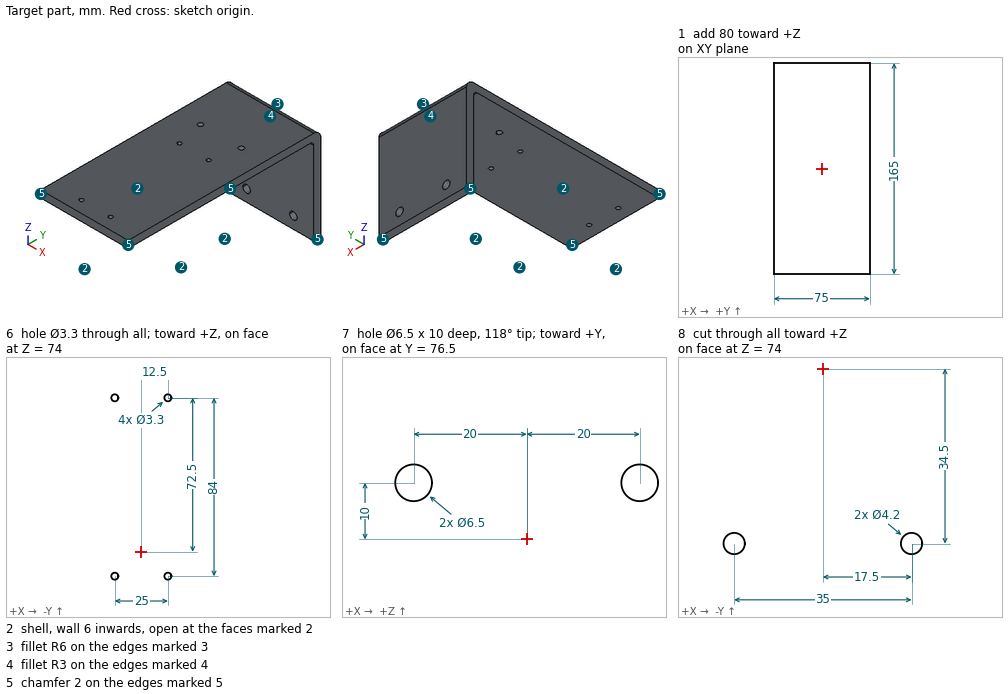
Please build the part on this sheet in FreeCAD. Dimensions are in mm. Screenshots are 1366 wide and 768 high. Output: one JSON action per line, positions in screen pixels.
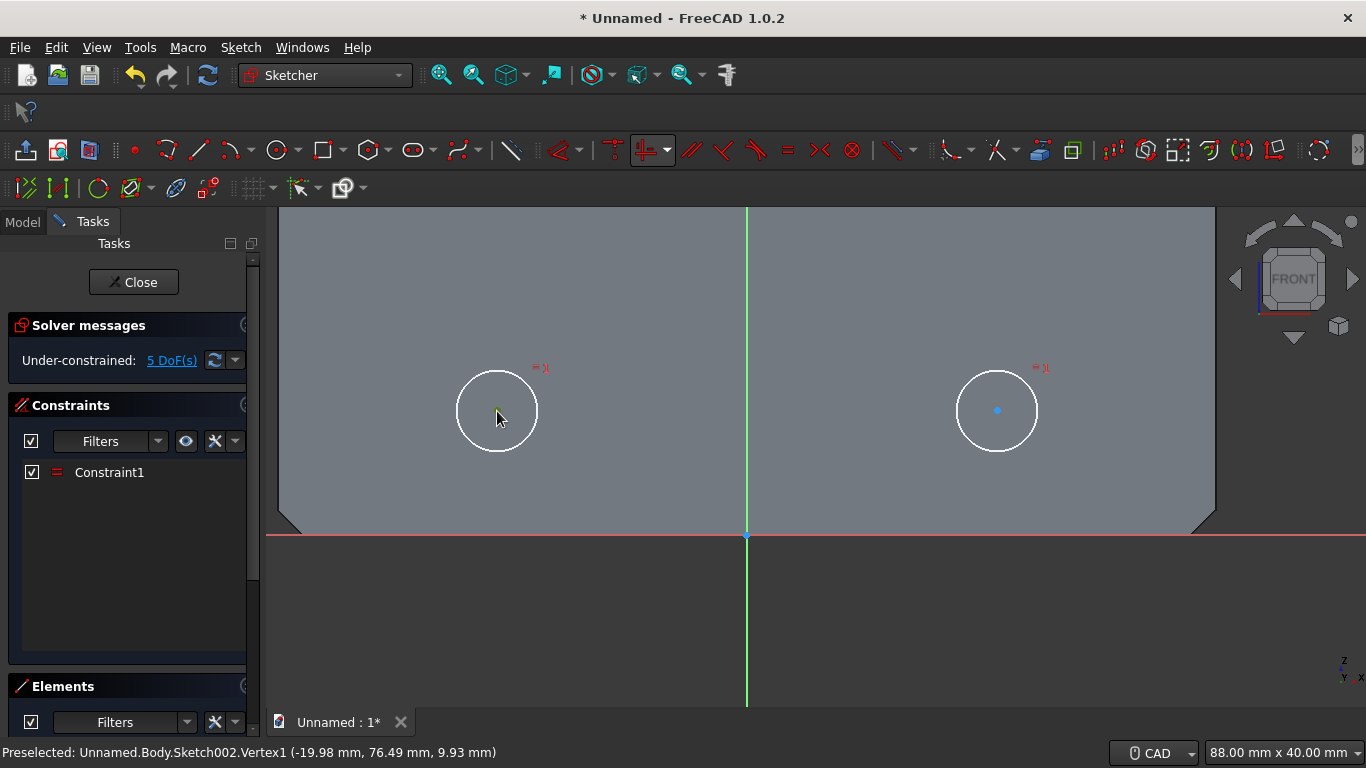
{"action": "left_click", "coordinate": [997, 411]}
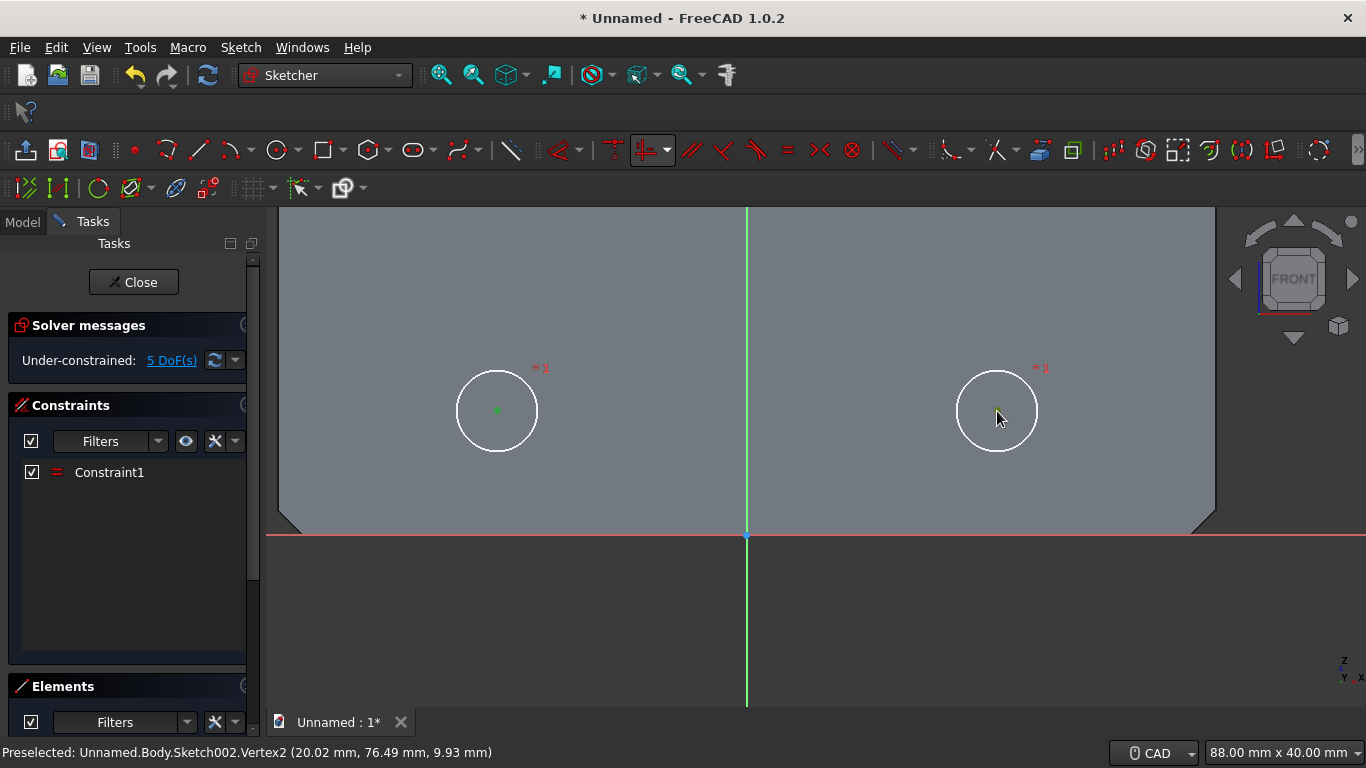
{"action": "left_click", "coordinate": [670, 150]}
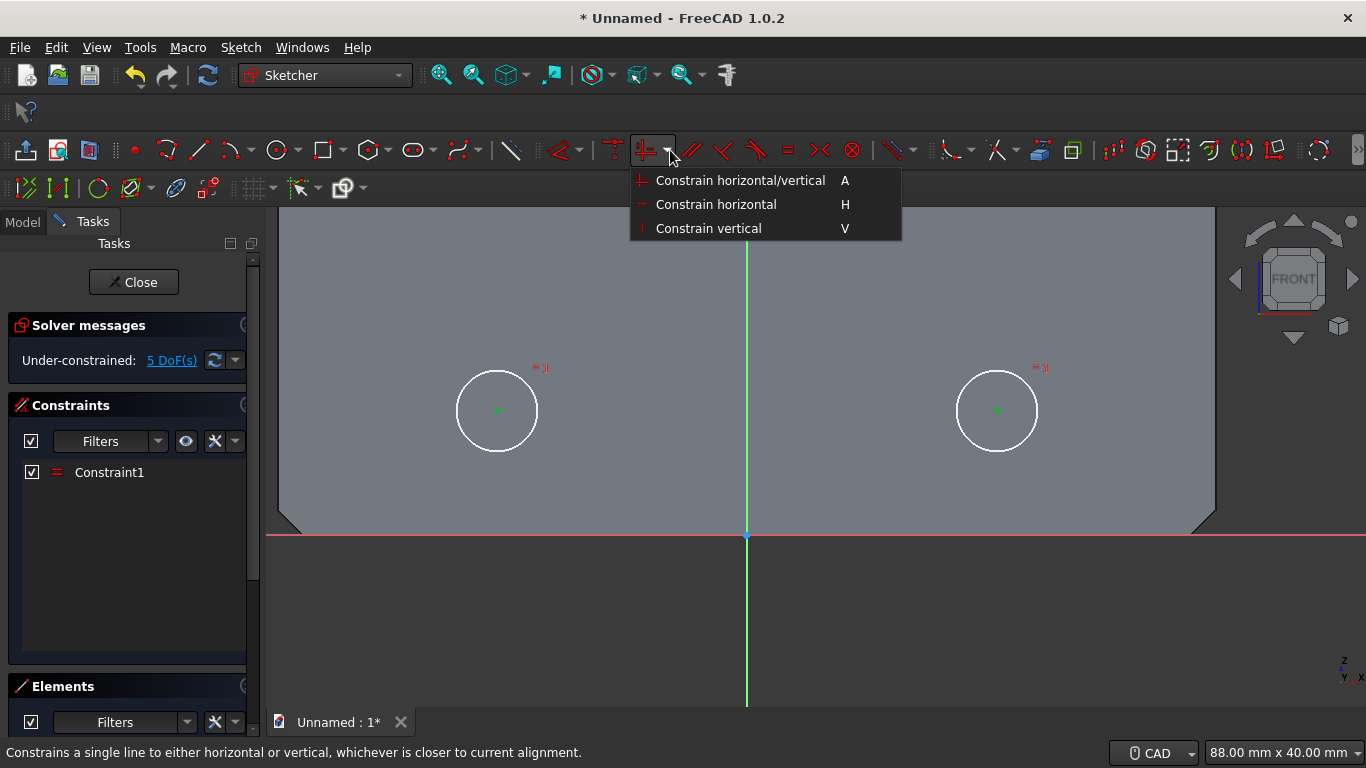
{"action": "left_click", "coordinate": [766, 204]}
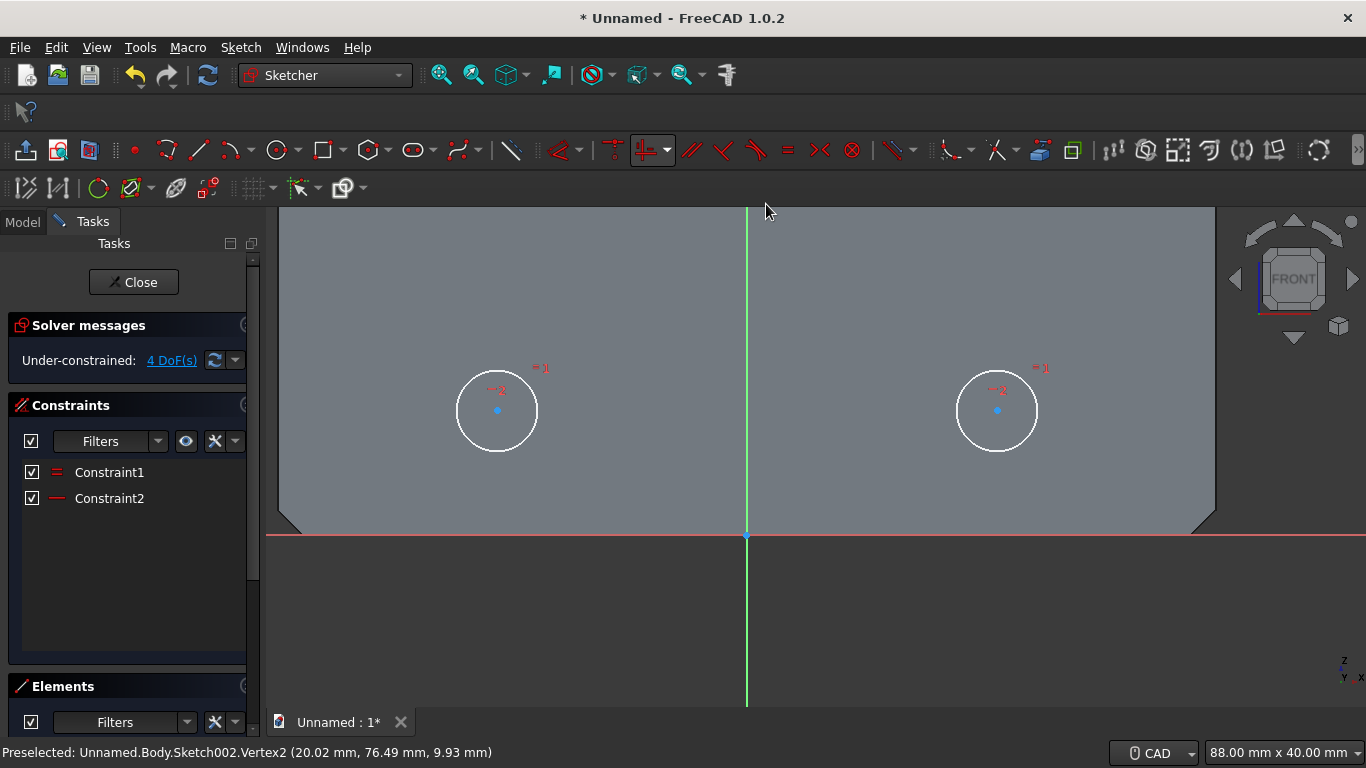
{"action": "left_click", "coordinate": [558, 150]}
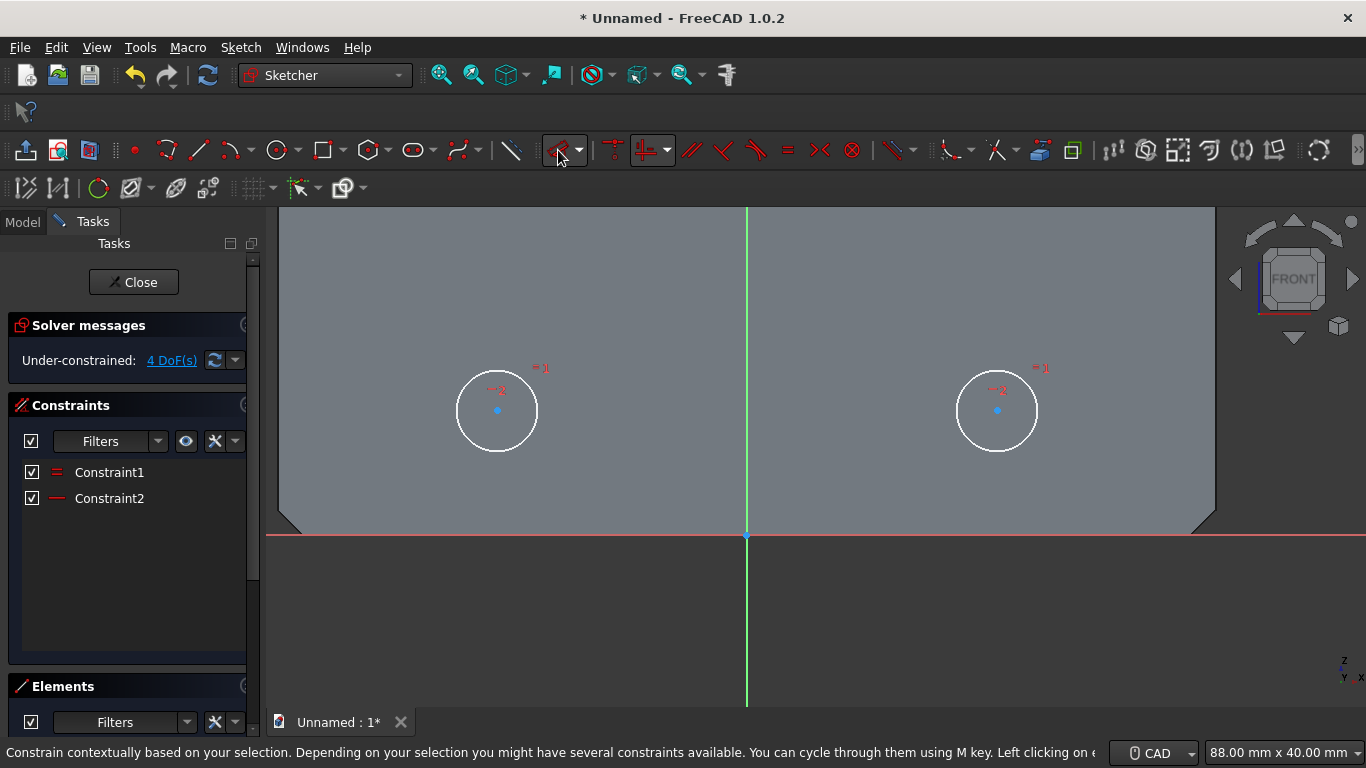
{"action": "left_click", "coordinate": [525, 382]}
{"action": "left_click", "coordinate": [547, 359]}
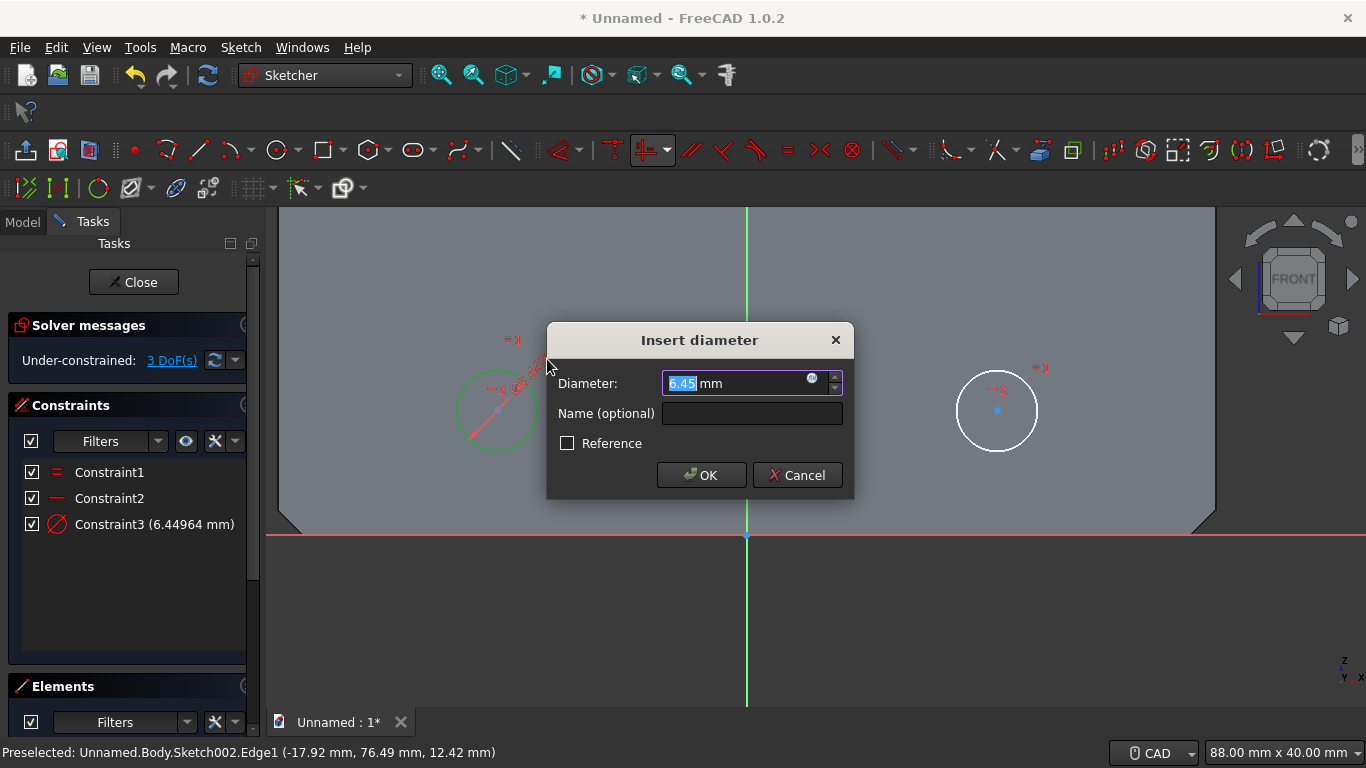
{"action": "type", "text": "6.5"}
{"action": "key", "text": "Return"}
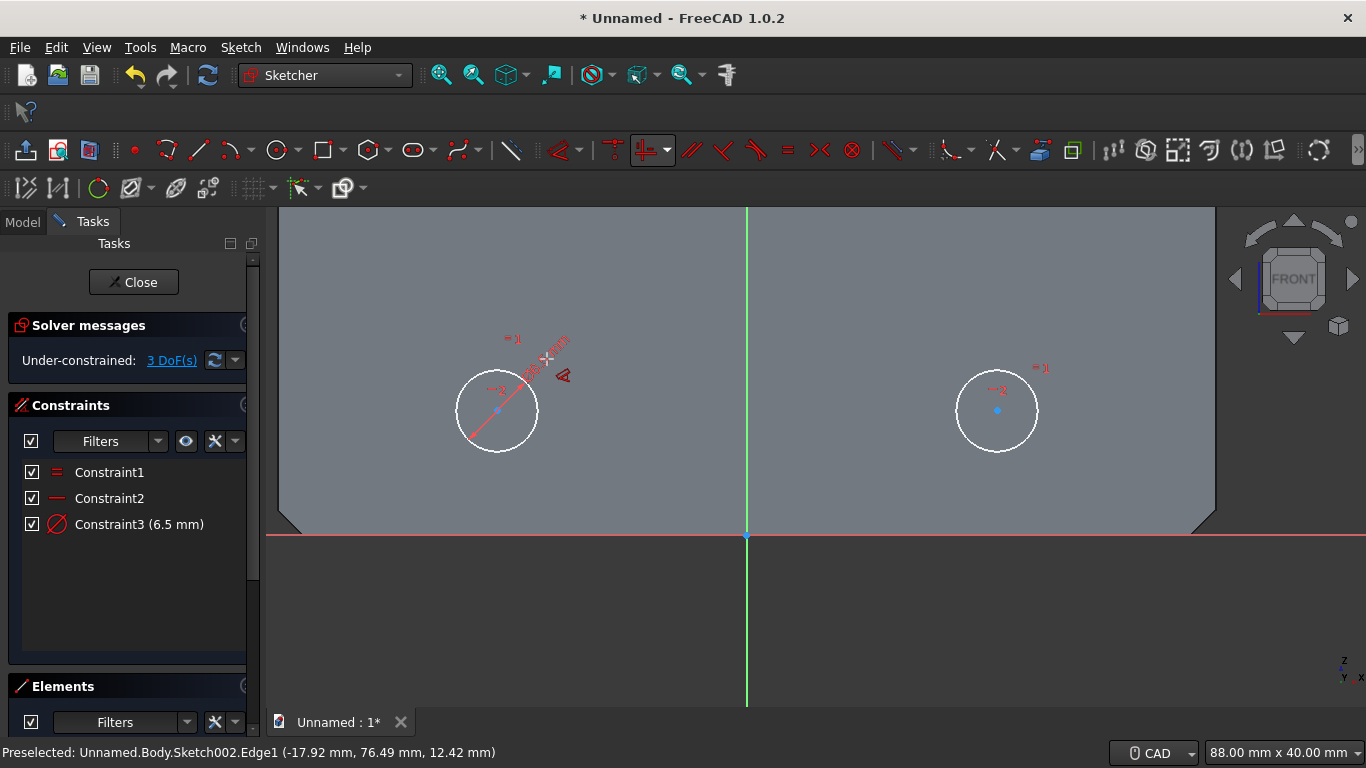
{"action": "left_click", "coordinate": [497, 411]}
{"action": "left_click", "coordinate": [622, 569]}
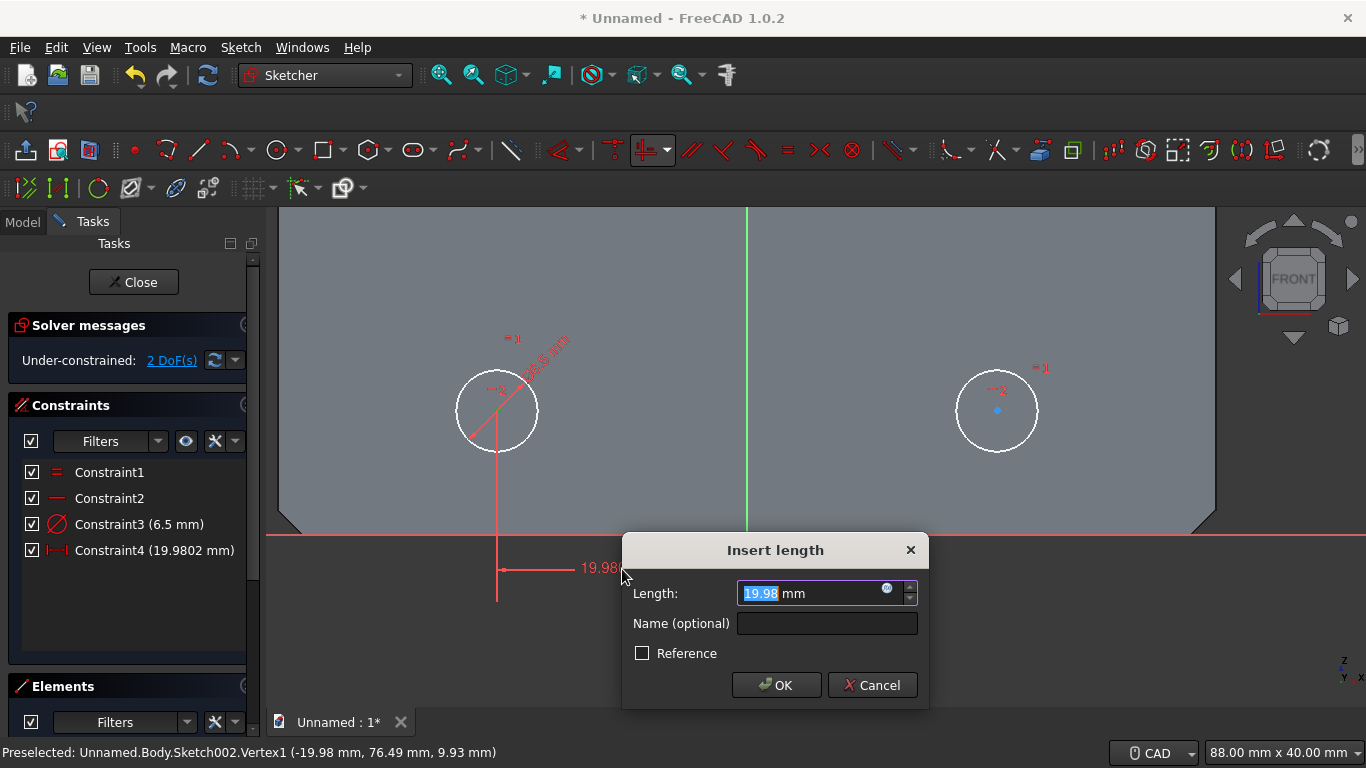
{"action": "type", "text": "20"}
{"action": "key", "text": "Return"}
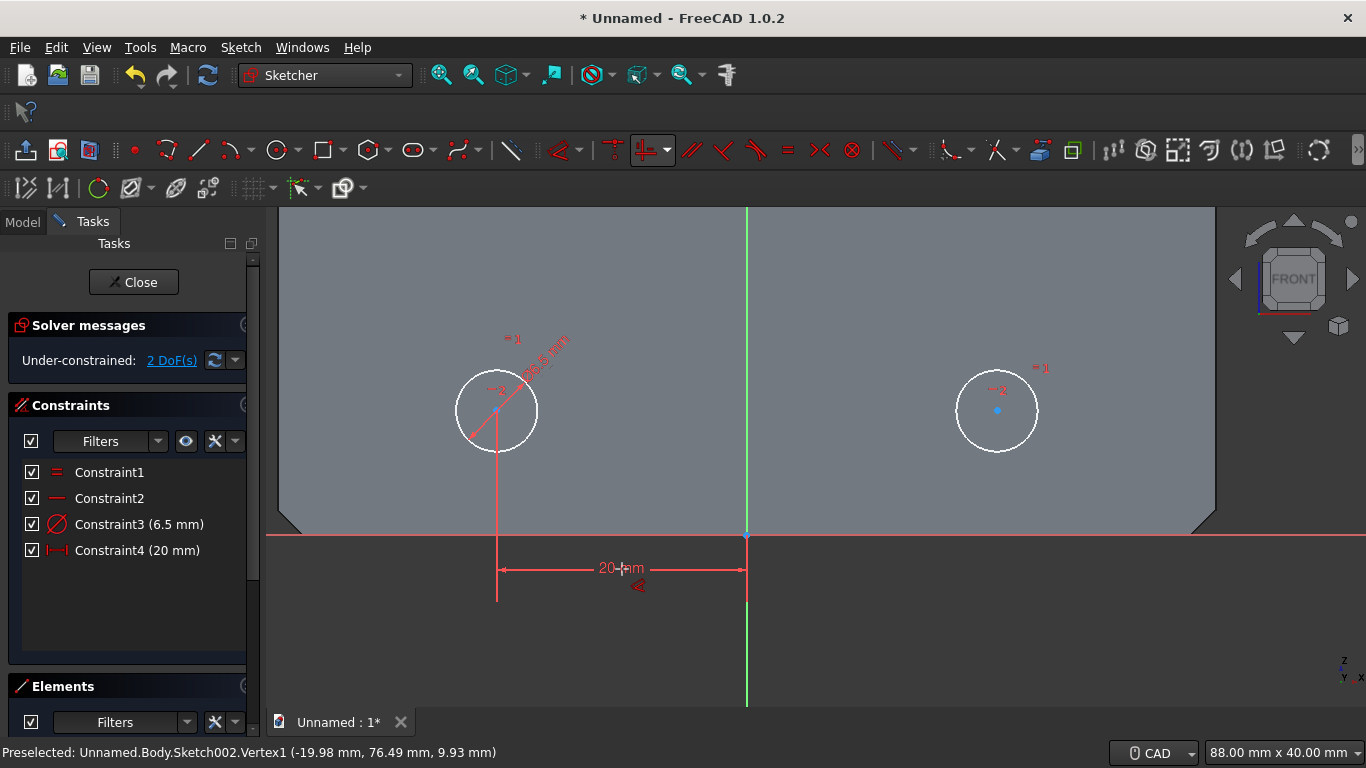
{"action": "left_click", "coordinate": [497, 411]}
{"action": "left_click", "coordinate": [463, 473]}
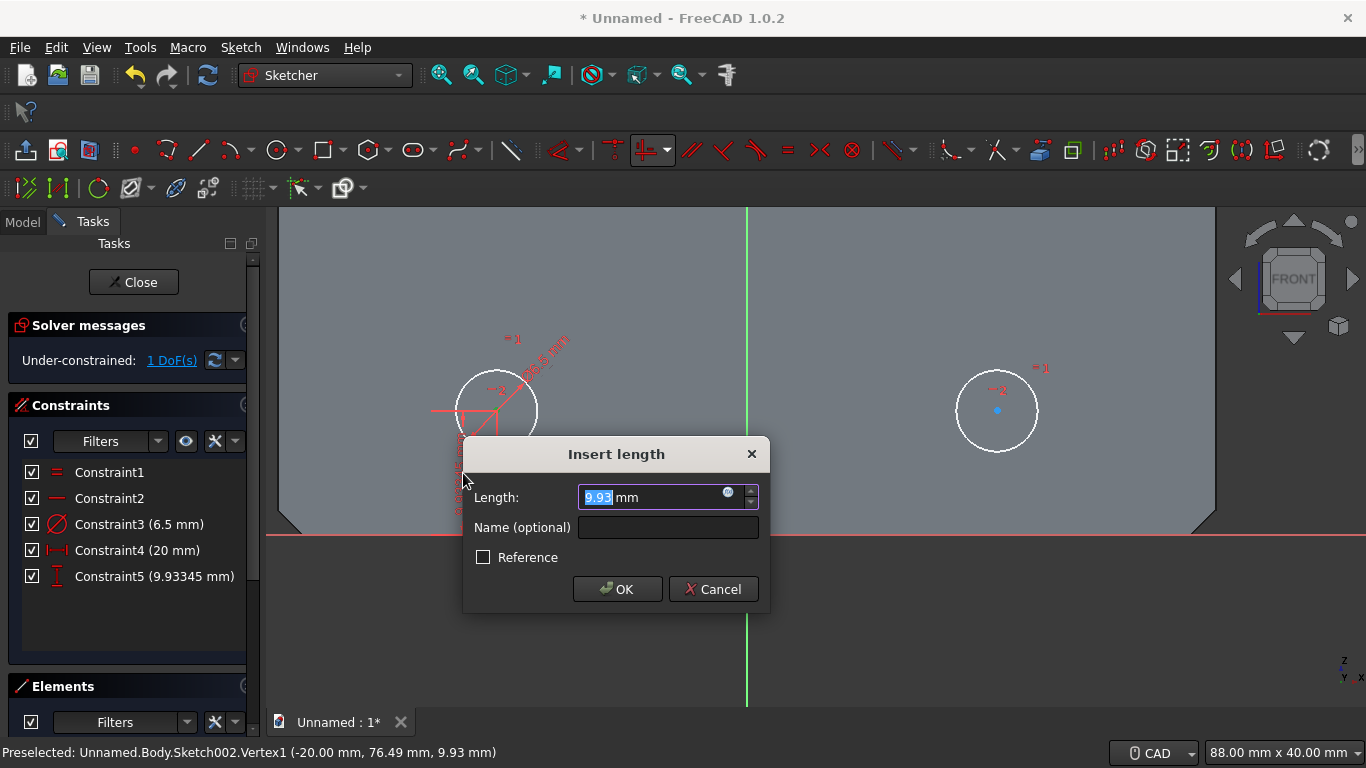
{"action": "type", "text": "10"}
{"action": "key", "text": "Return"}